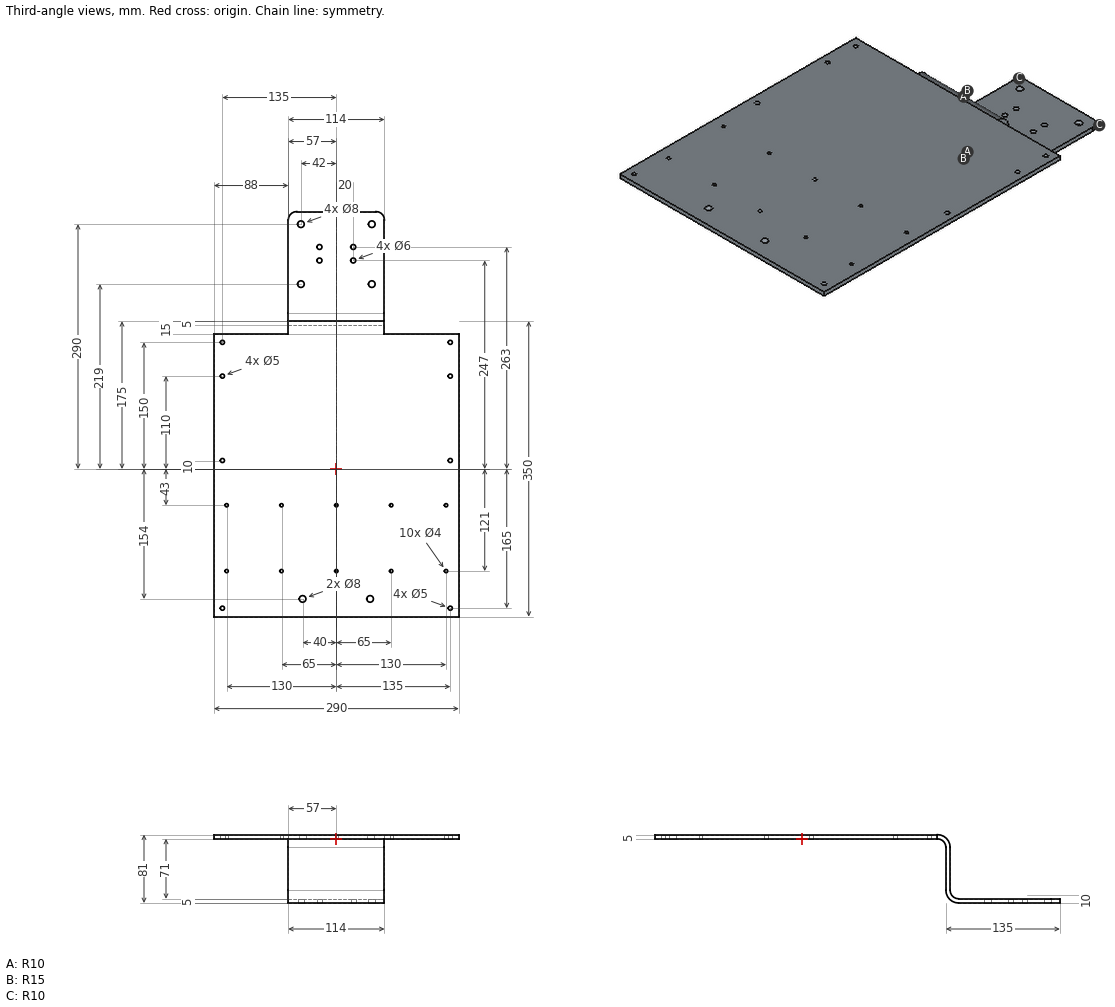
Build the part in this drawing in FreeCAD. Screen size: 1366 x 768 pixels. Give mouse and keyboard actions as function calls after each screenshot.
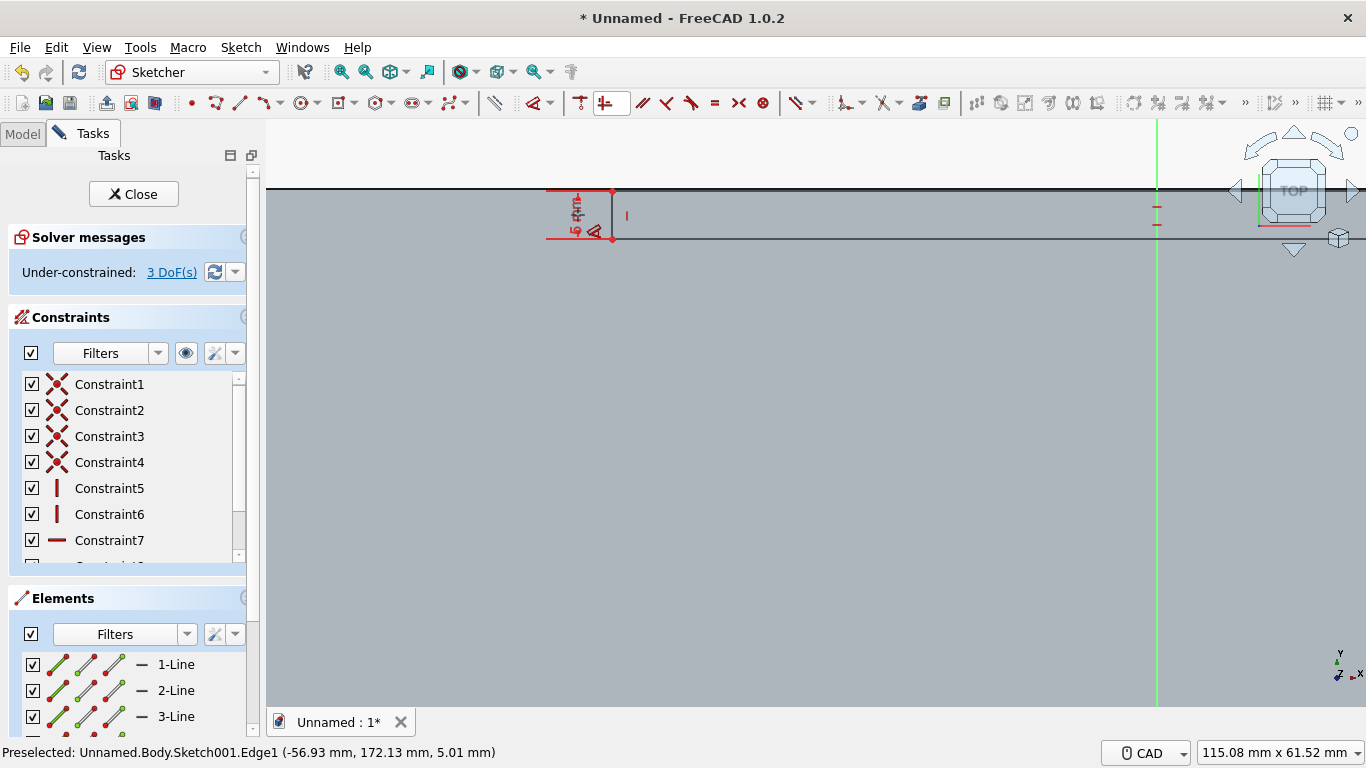
scroll(614, 213, down, 7)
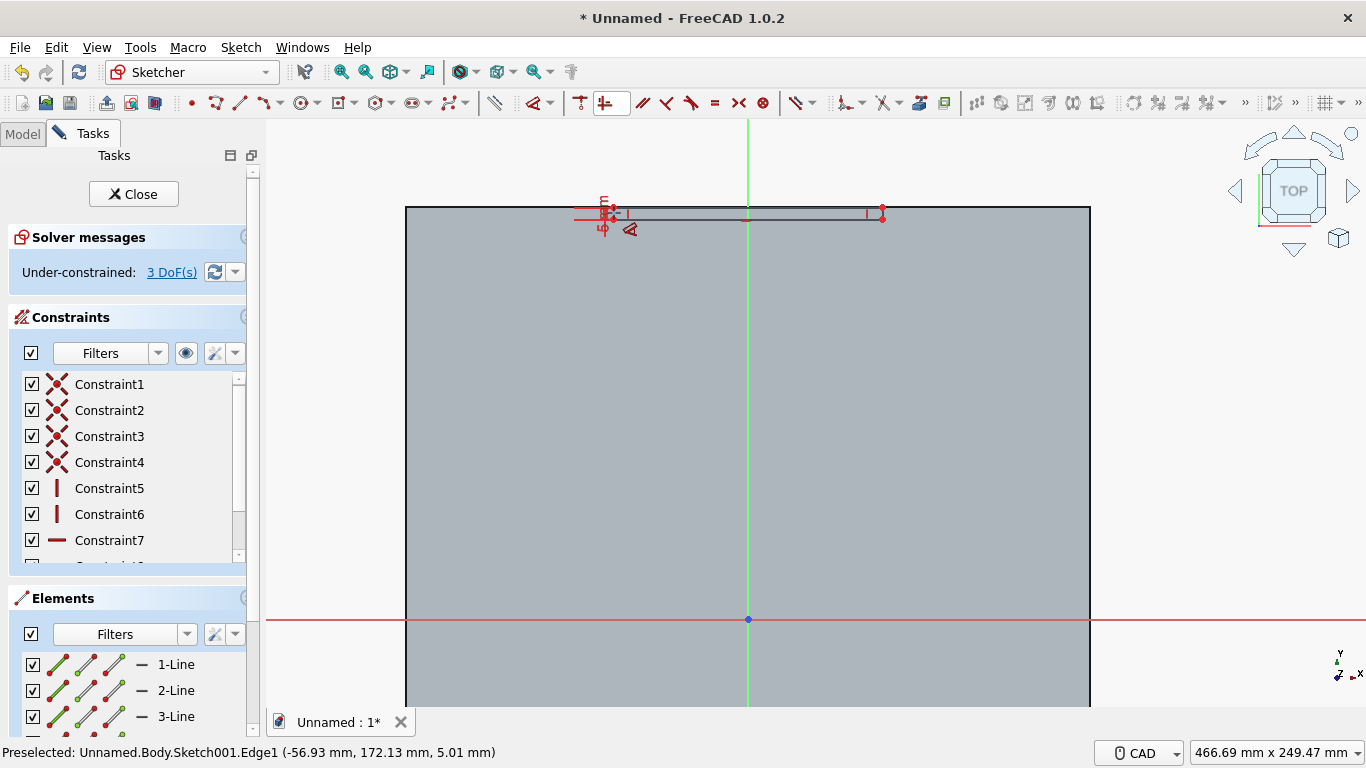
click(694, 220)
click(686, 186)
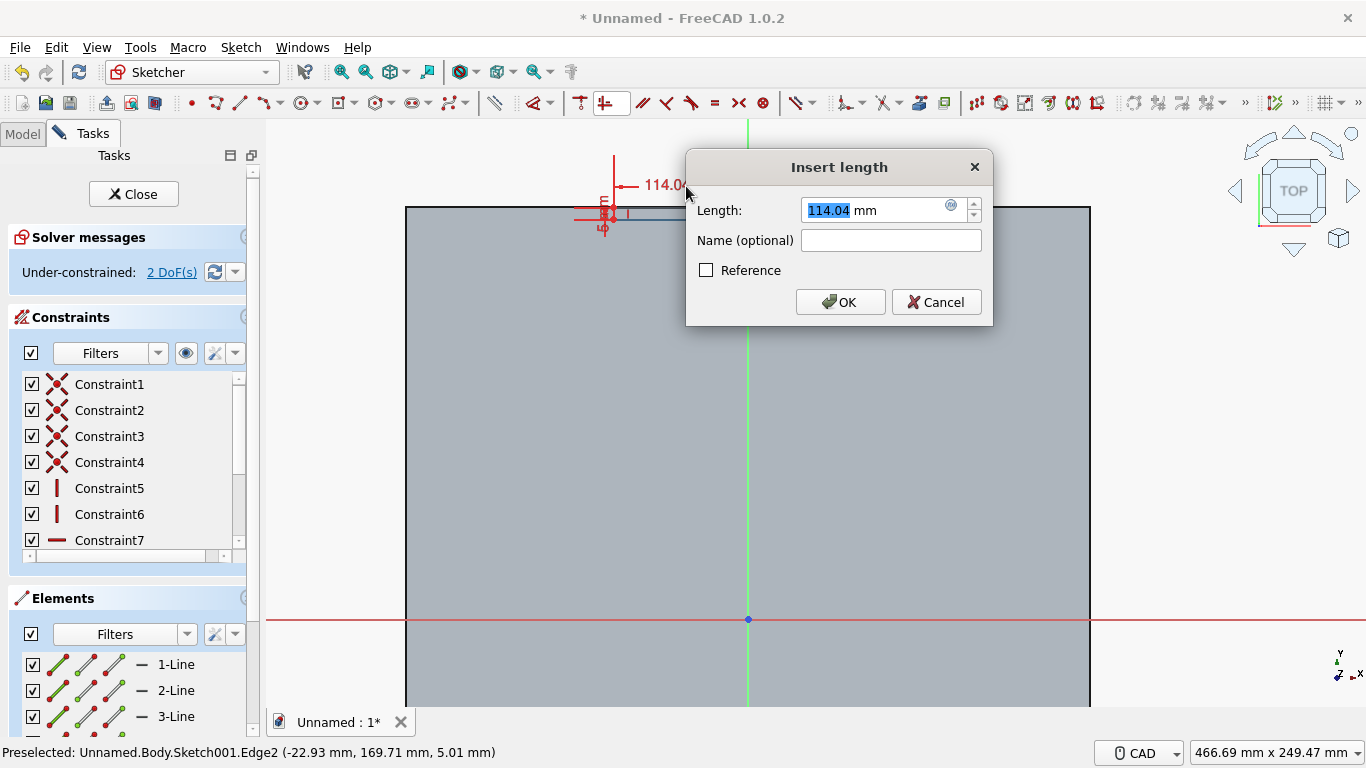
text(114)
key(Return)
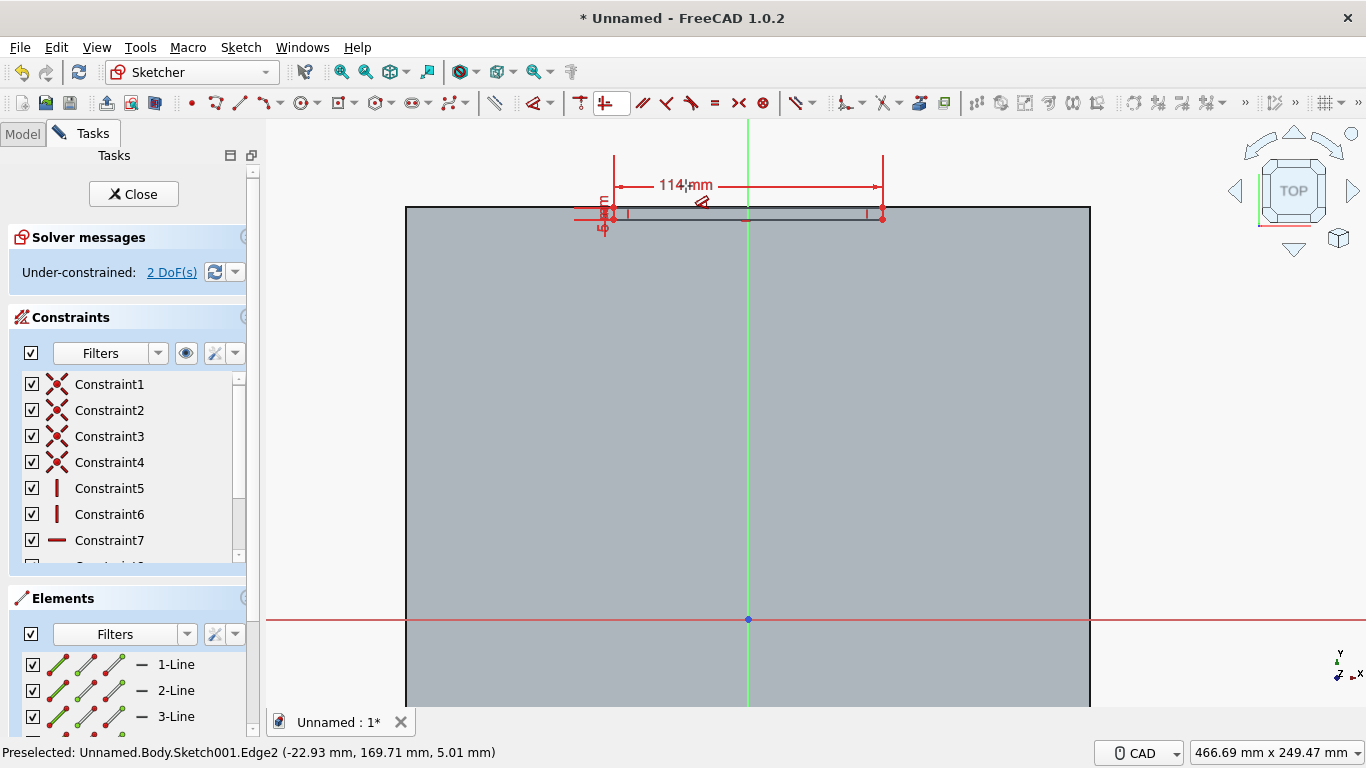
click(614, 208)
click(681, 654)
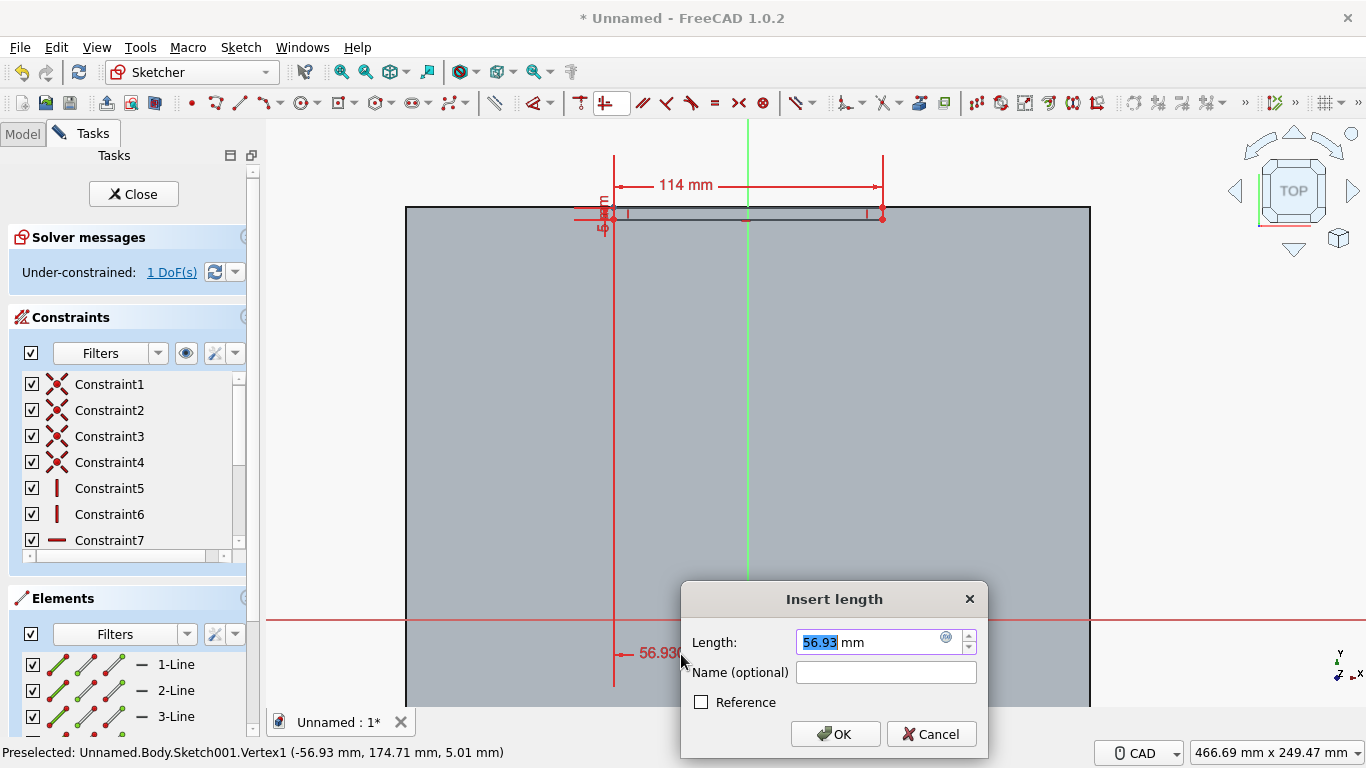
text(57)
key(Return)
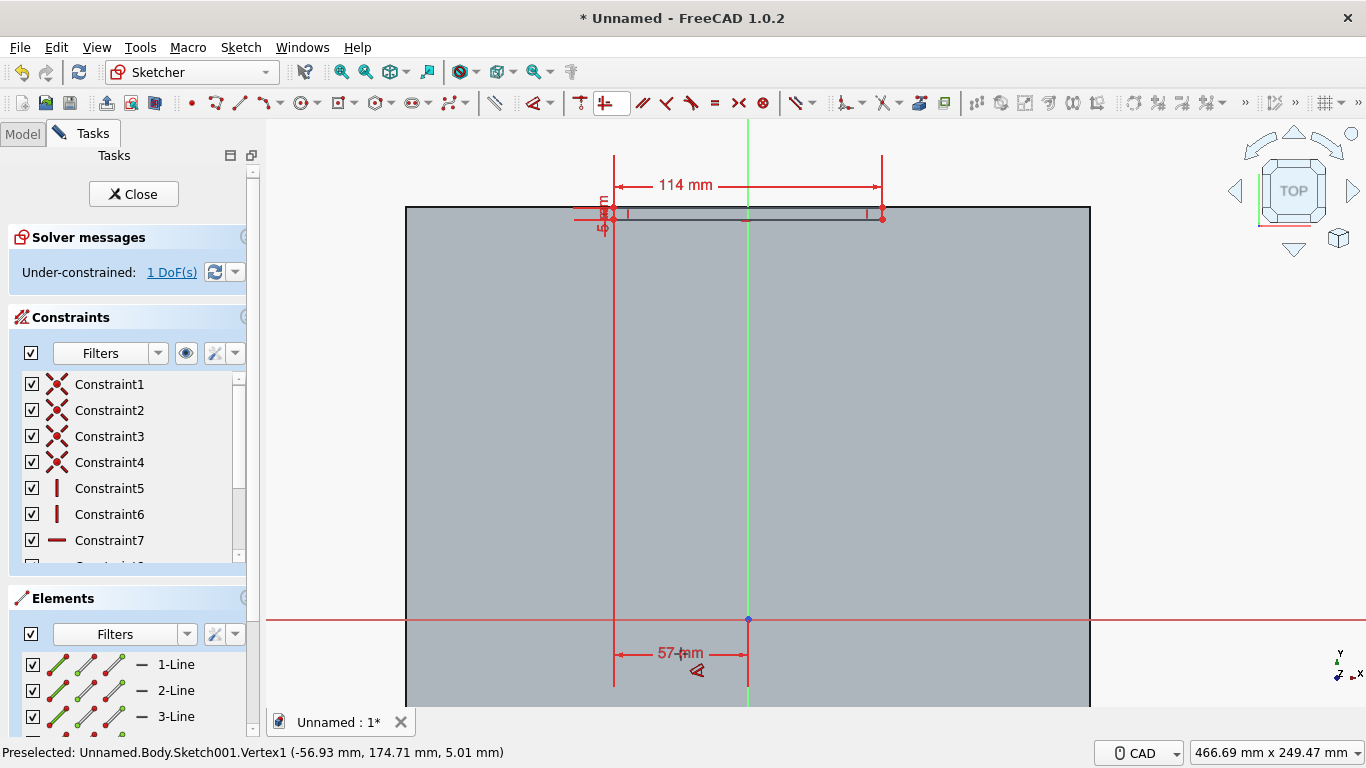
click(614, 208)
click(580, 414)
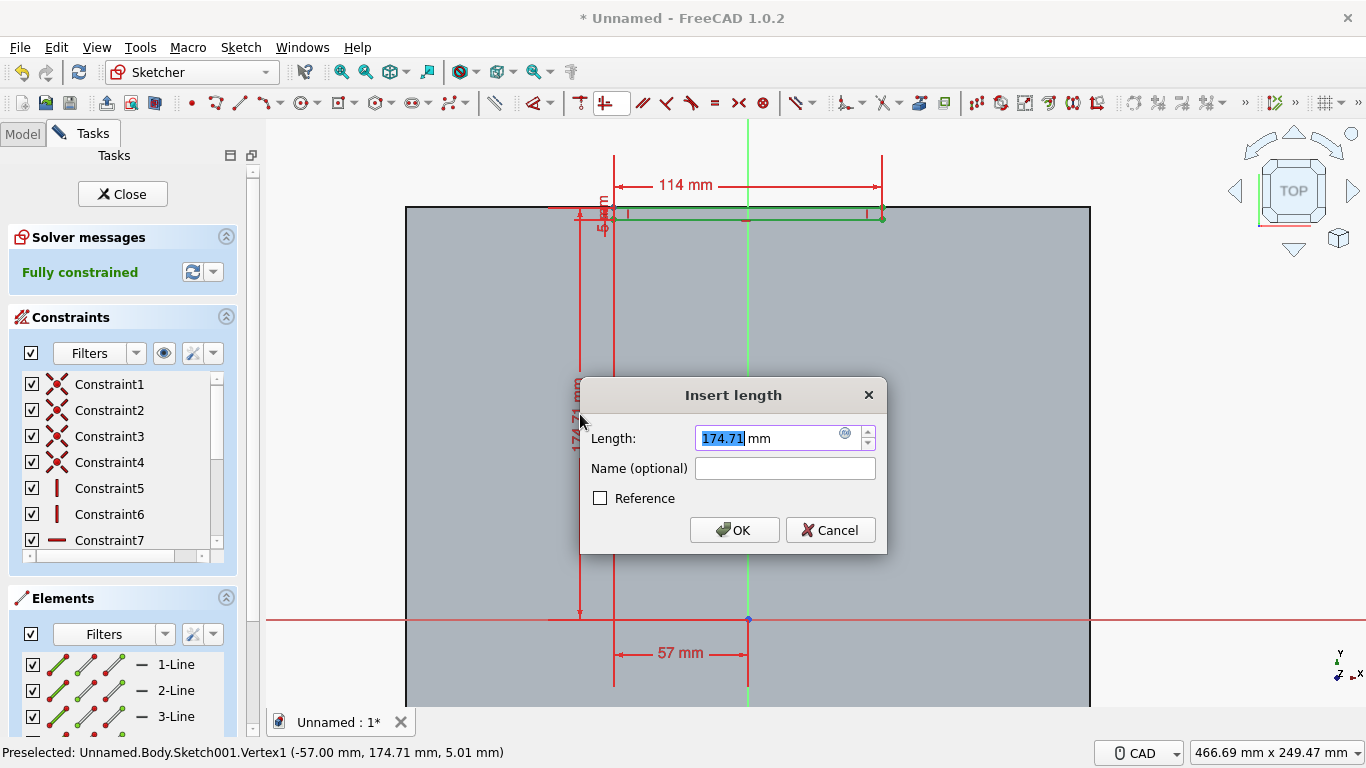
text(175)
key(Return)
key(Escape)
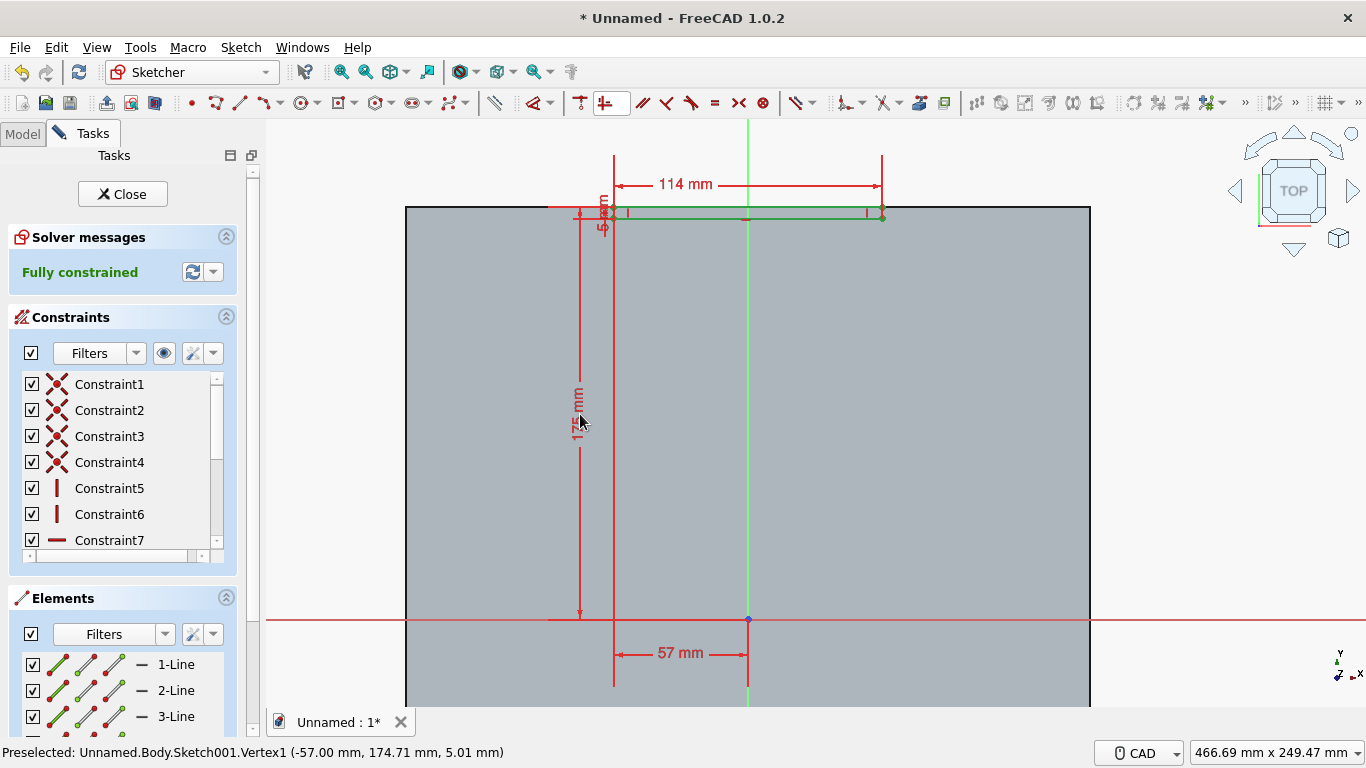
click(123, 194)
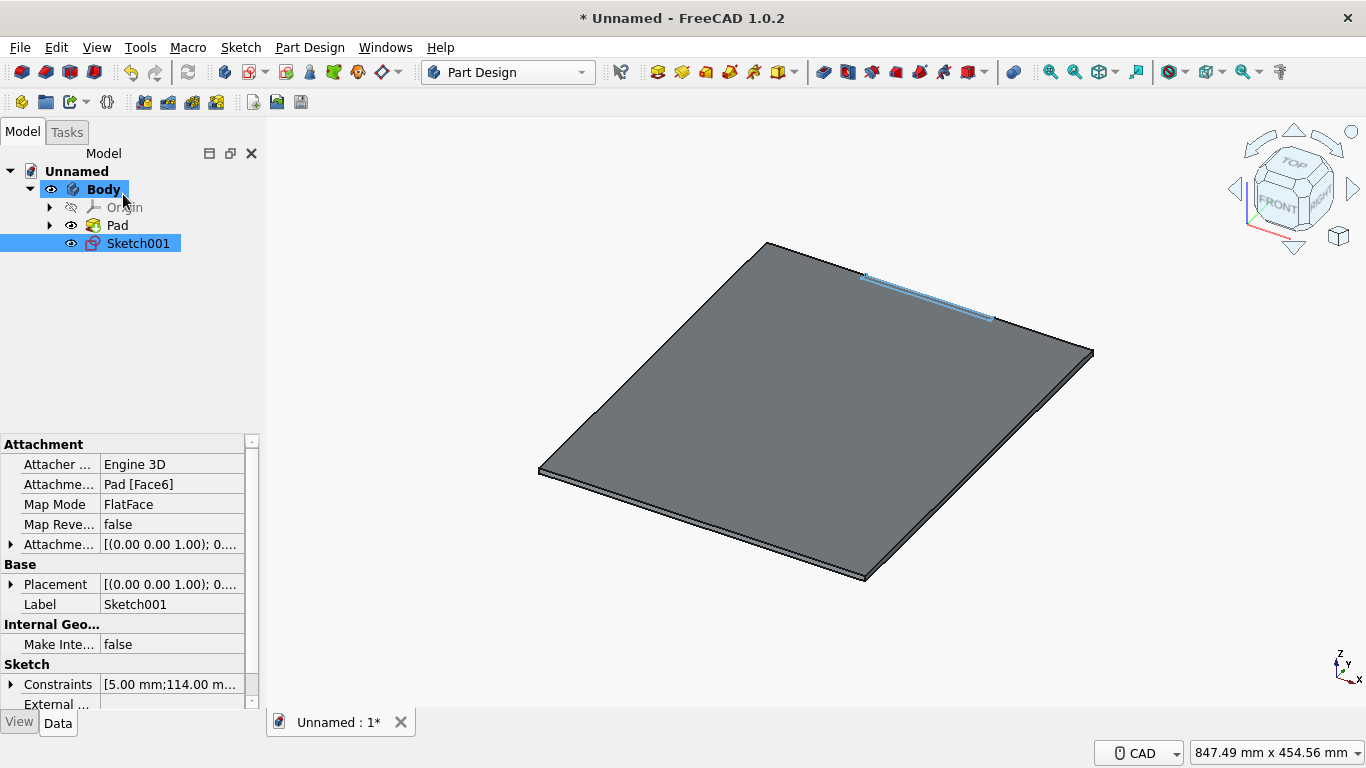
click(658, 72)